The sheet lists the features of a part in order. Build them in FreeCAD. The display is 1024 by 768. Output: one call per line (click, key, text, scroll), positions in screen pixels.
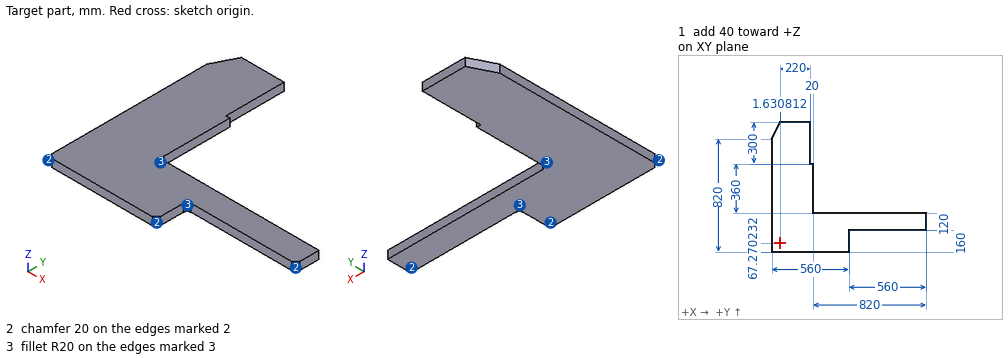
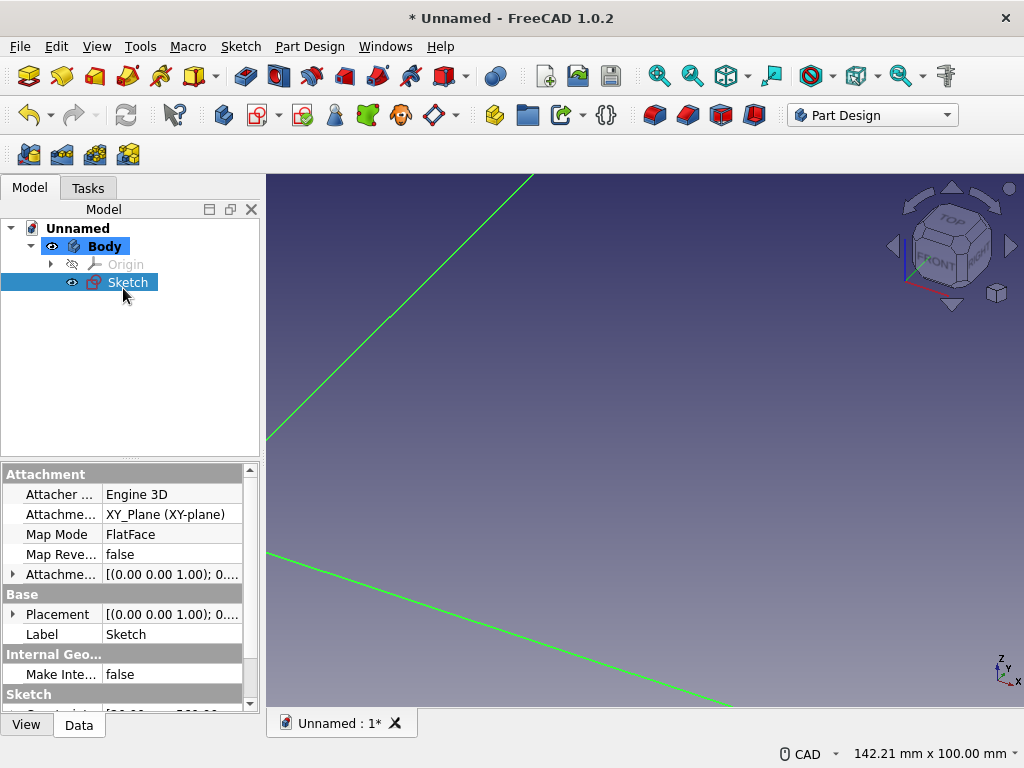
click(29, 76)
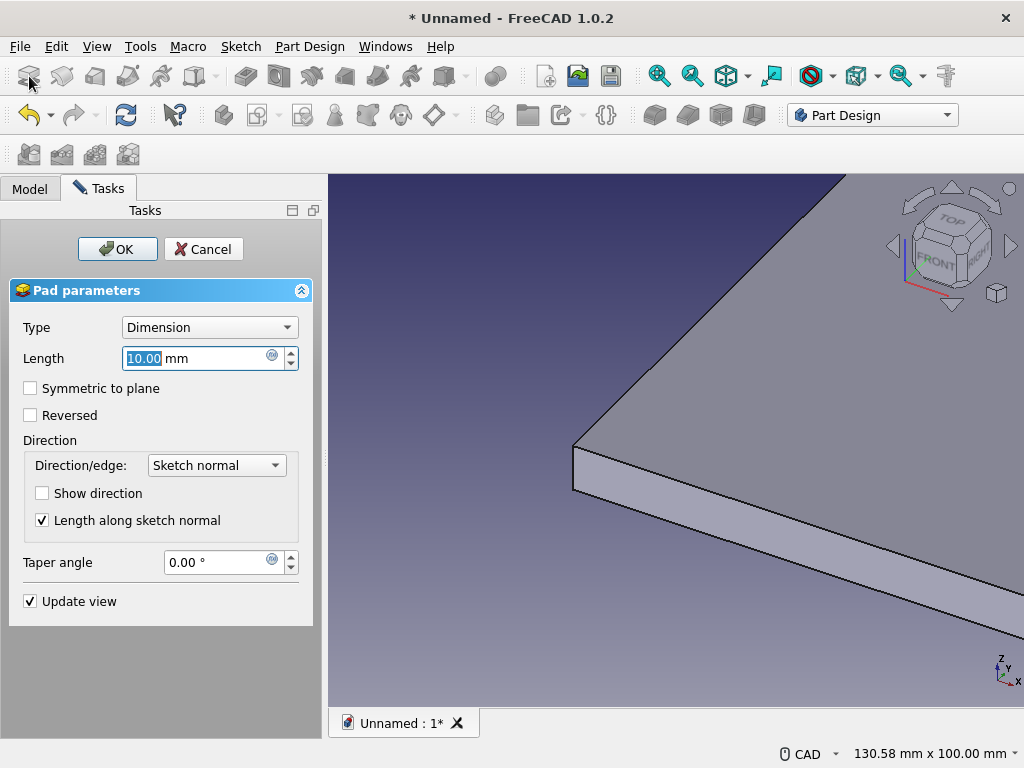
text(40)
key(Tab)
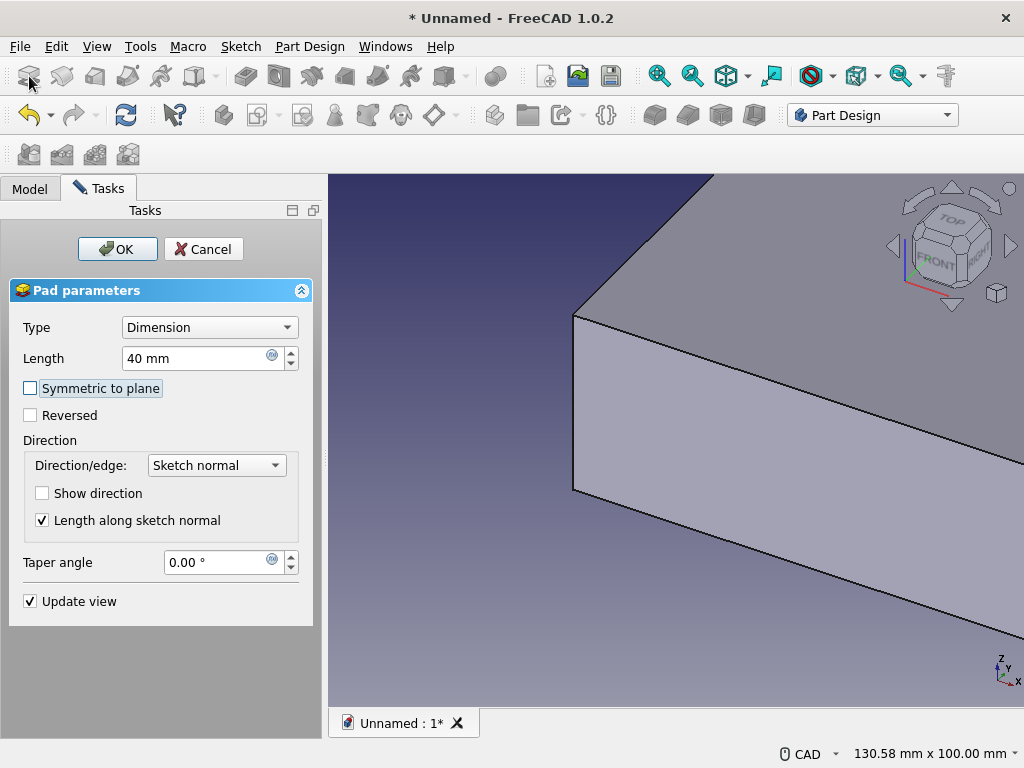
click(118, 249)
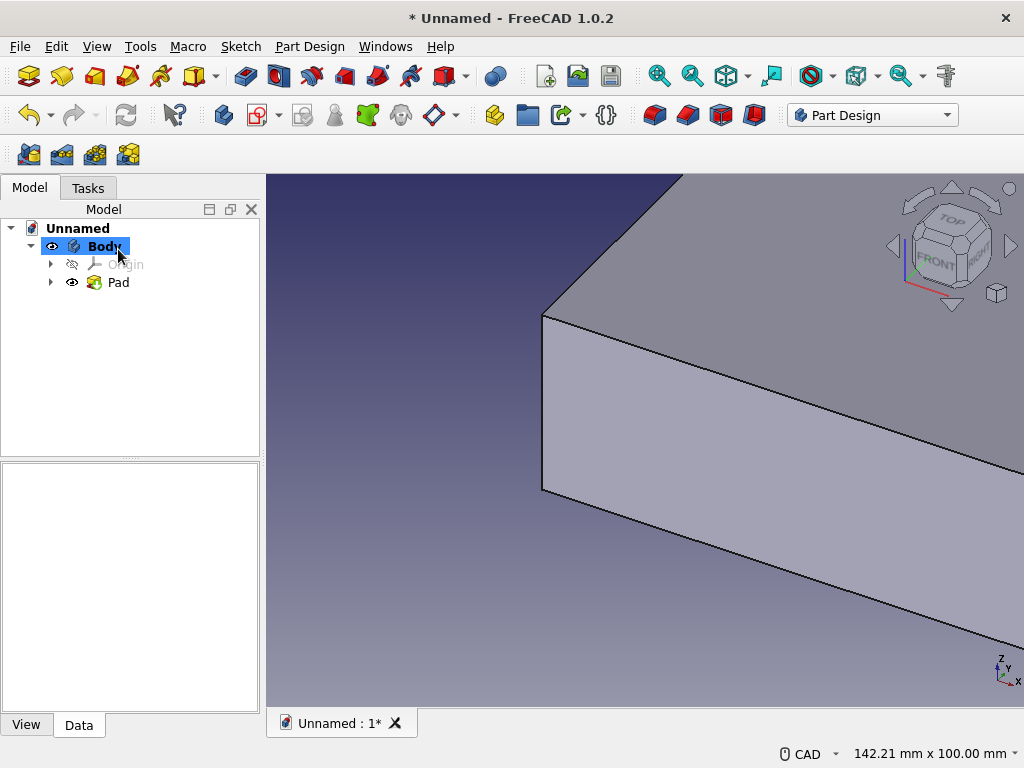
key(v)
key(f)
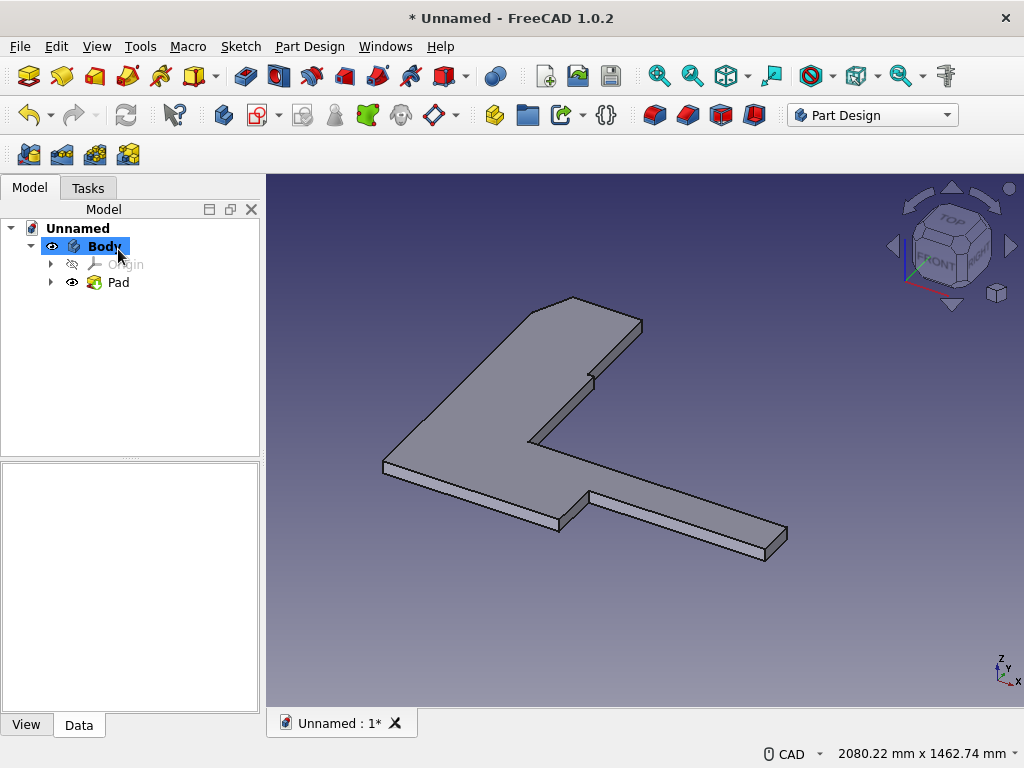
click(765, 555)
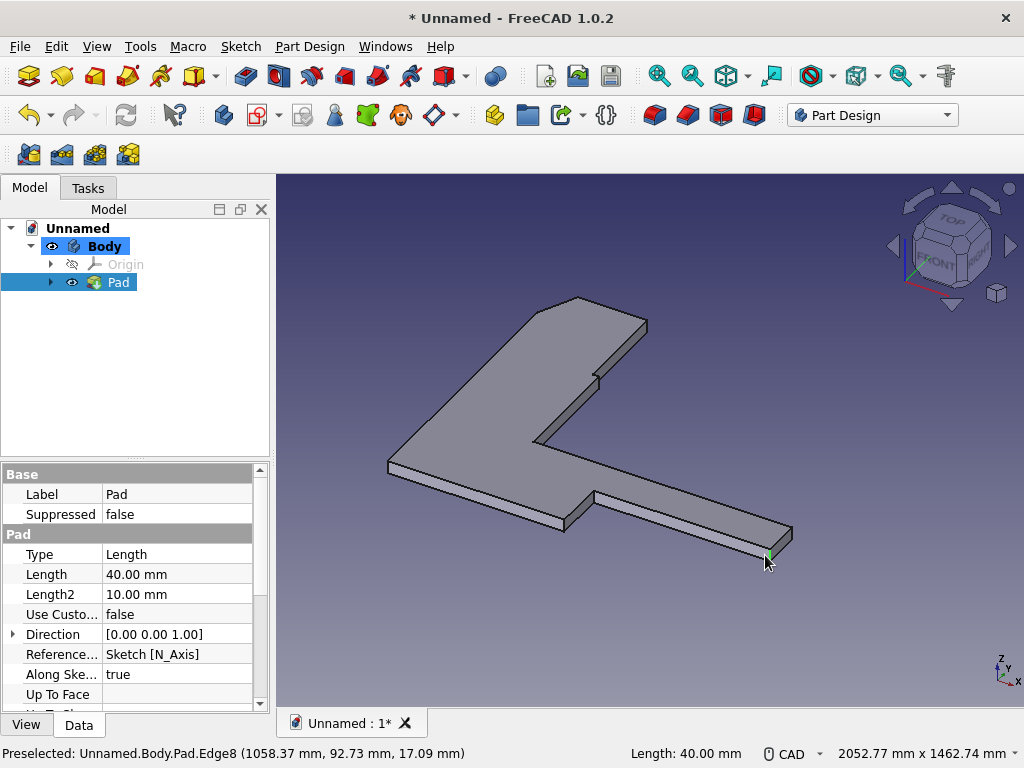
click(564, 525, ctrl)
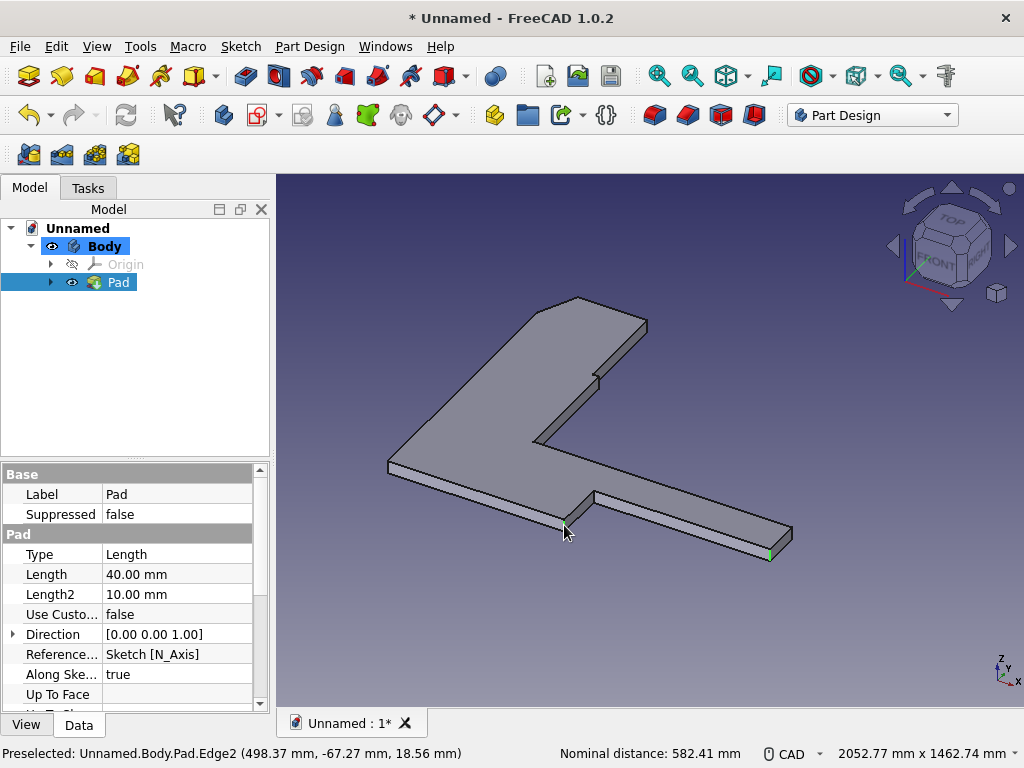
scroll(388, 466, up, 6)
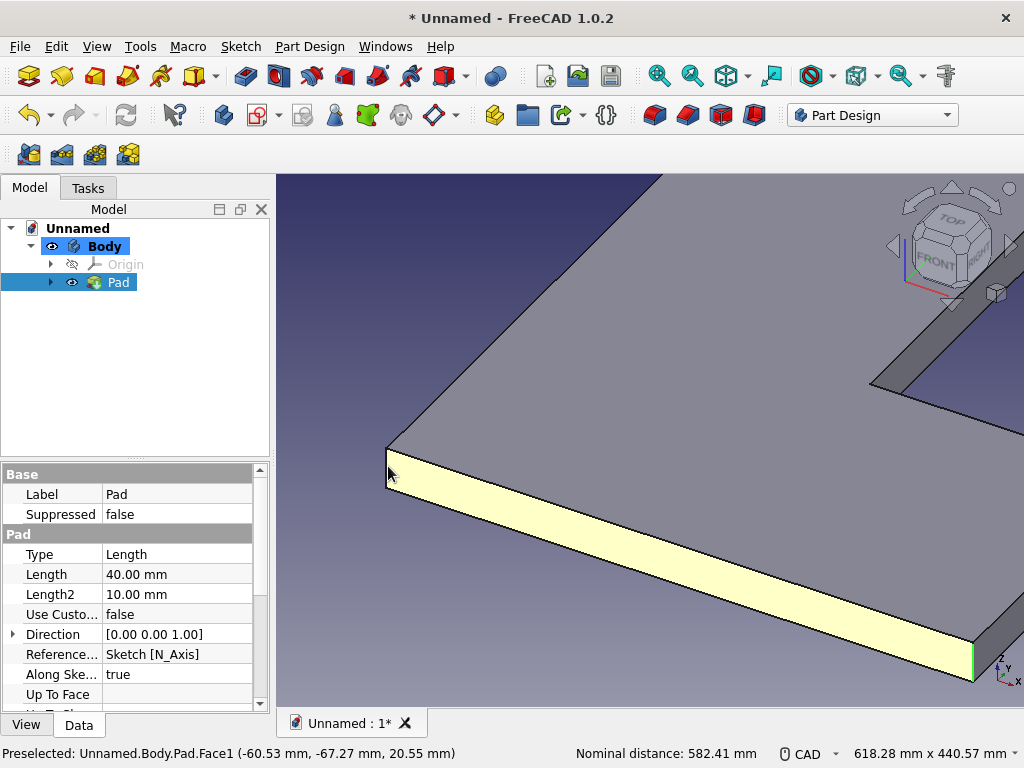
key(v)
key(f)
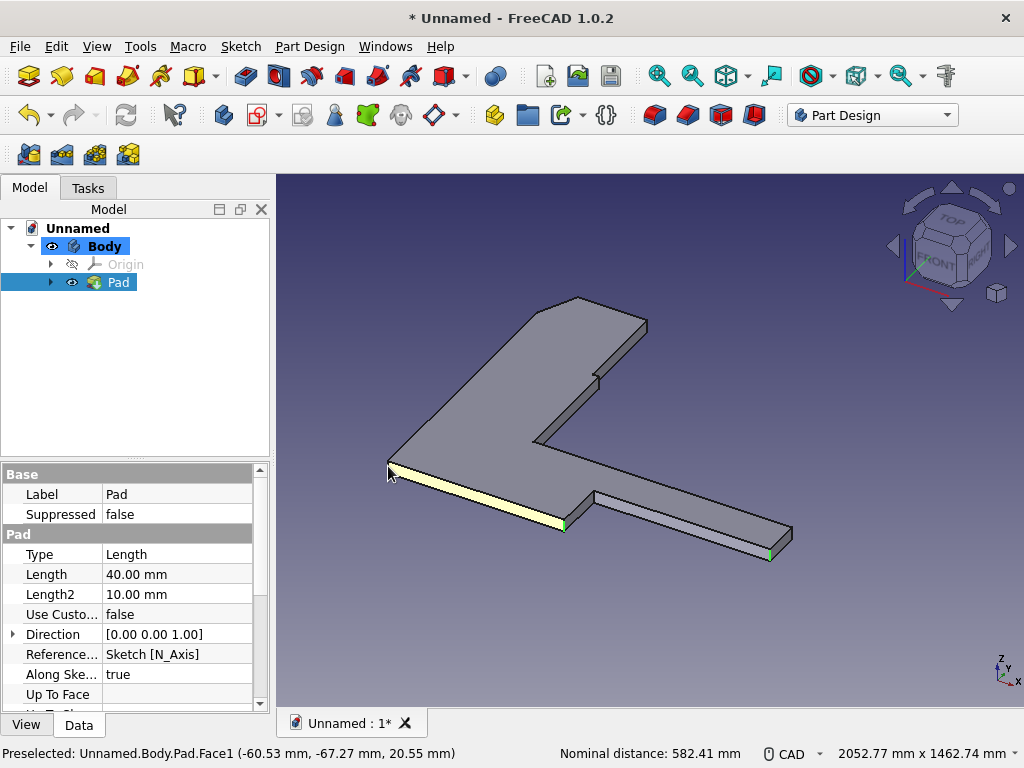
key(0)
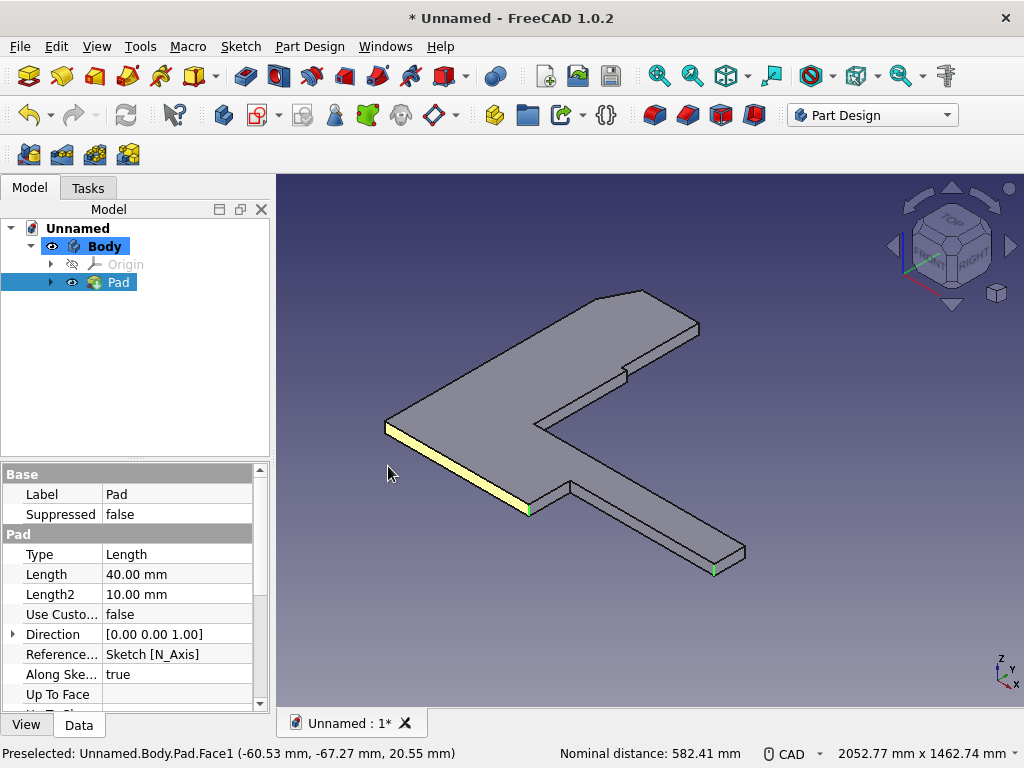
scroll(385, 426, up, 6)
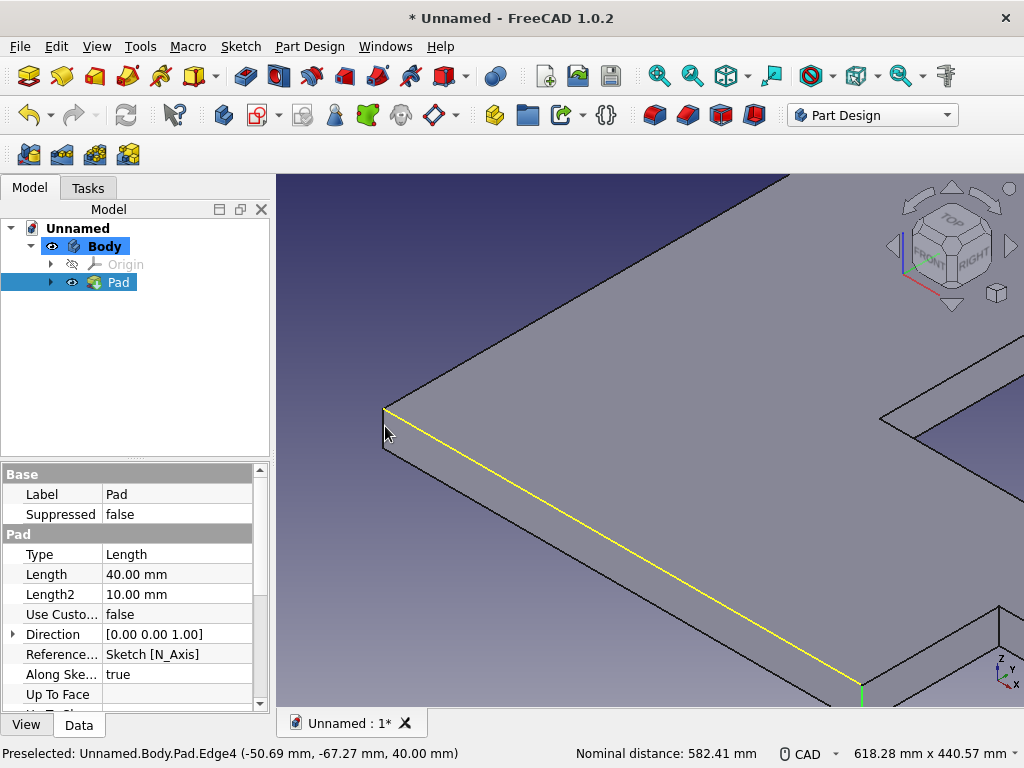
key(v)
key(f)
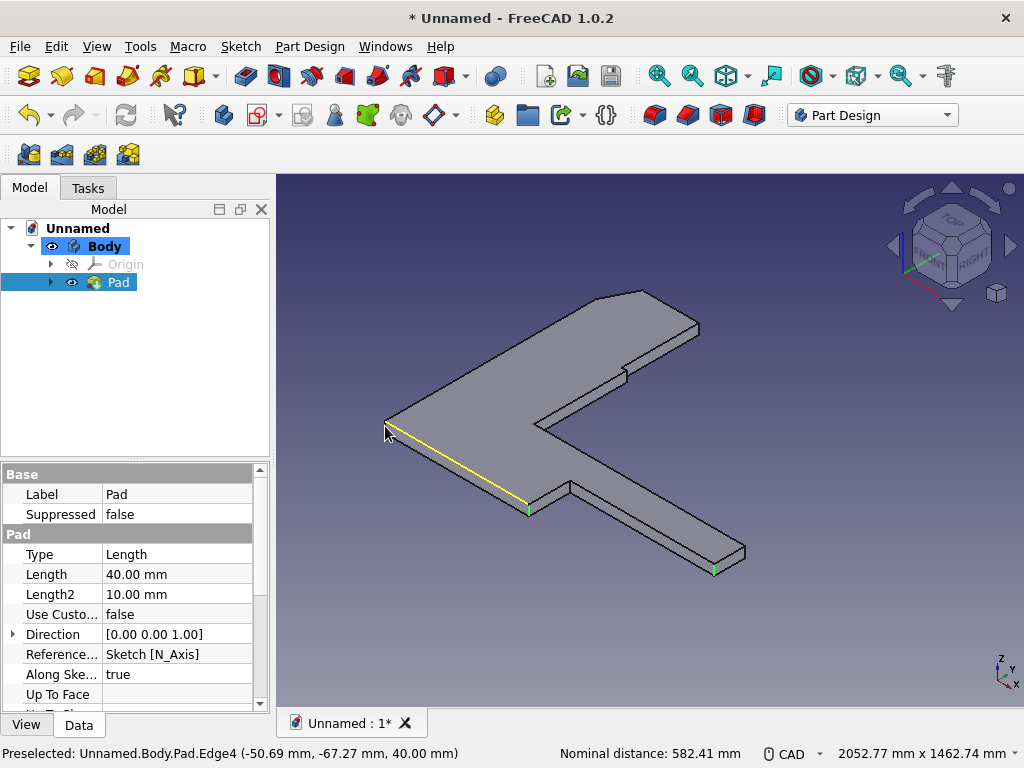
key(2)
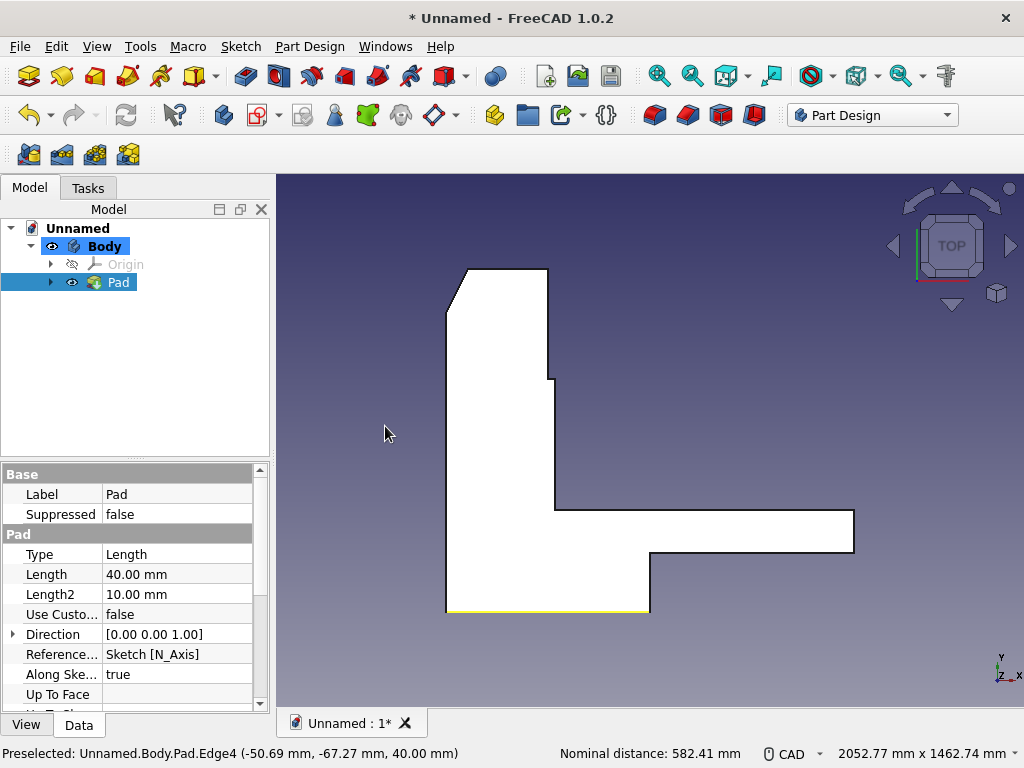
scroll(446, 611, up, 6)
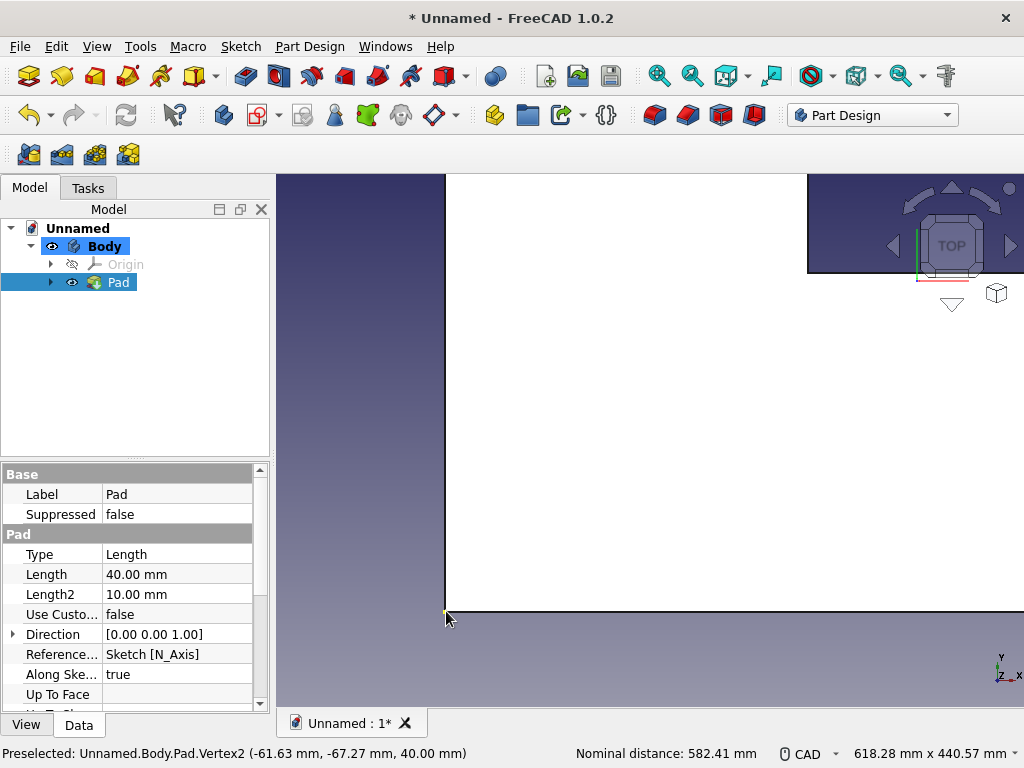
key(v)
key(f)